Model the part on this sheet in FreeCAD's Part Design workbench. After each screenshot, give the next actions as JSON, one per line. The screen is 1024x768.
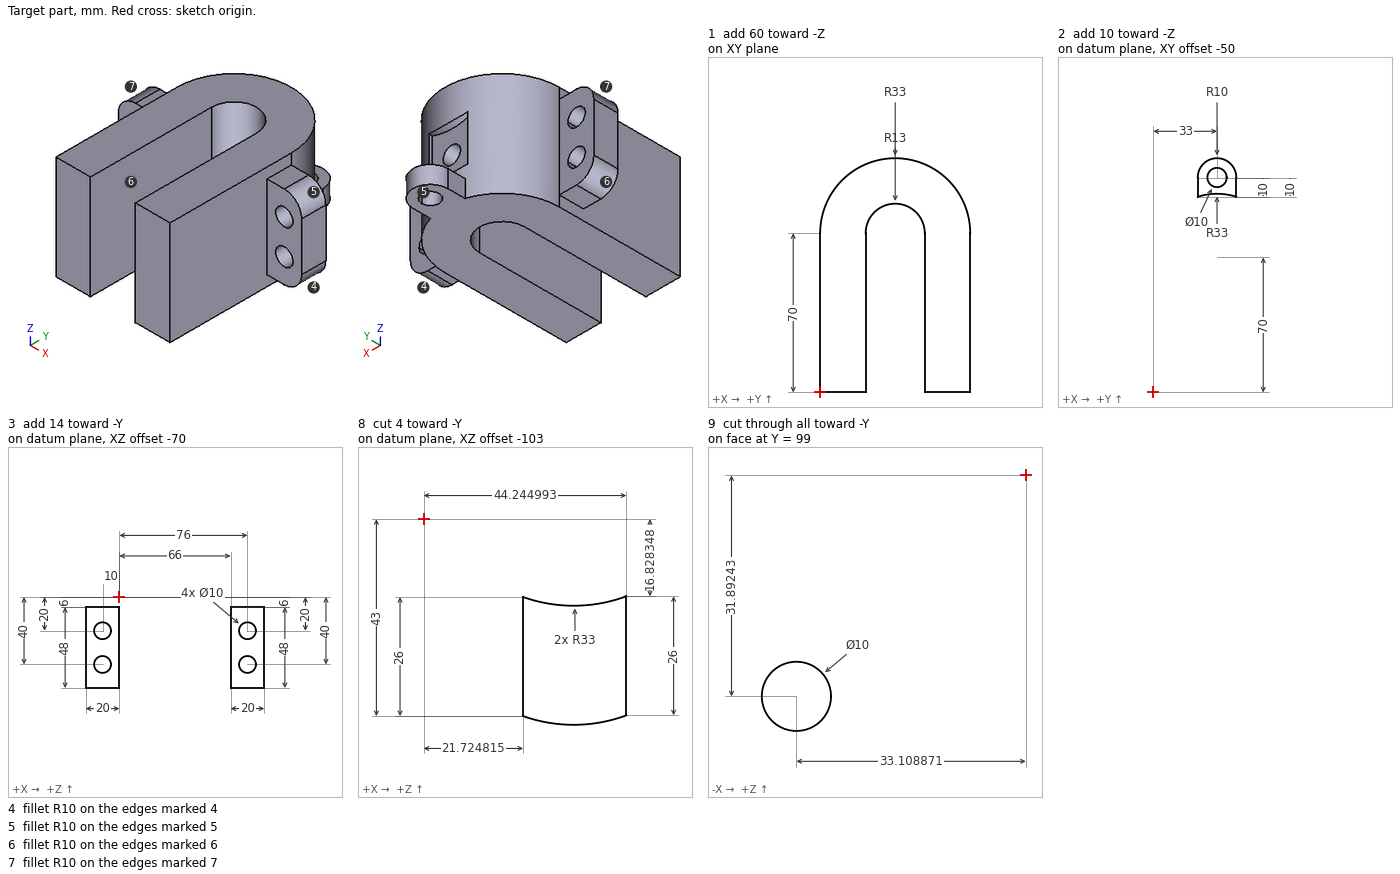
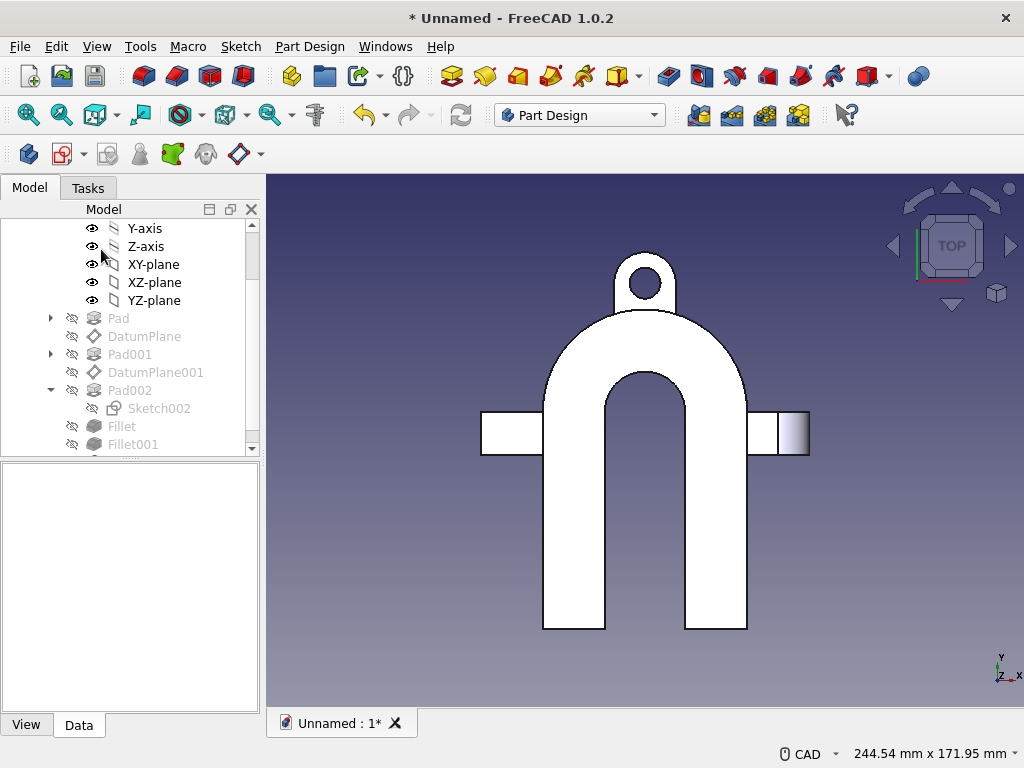
{"action": "left_click", "coordinate": [481, 432]}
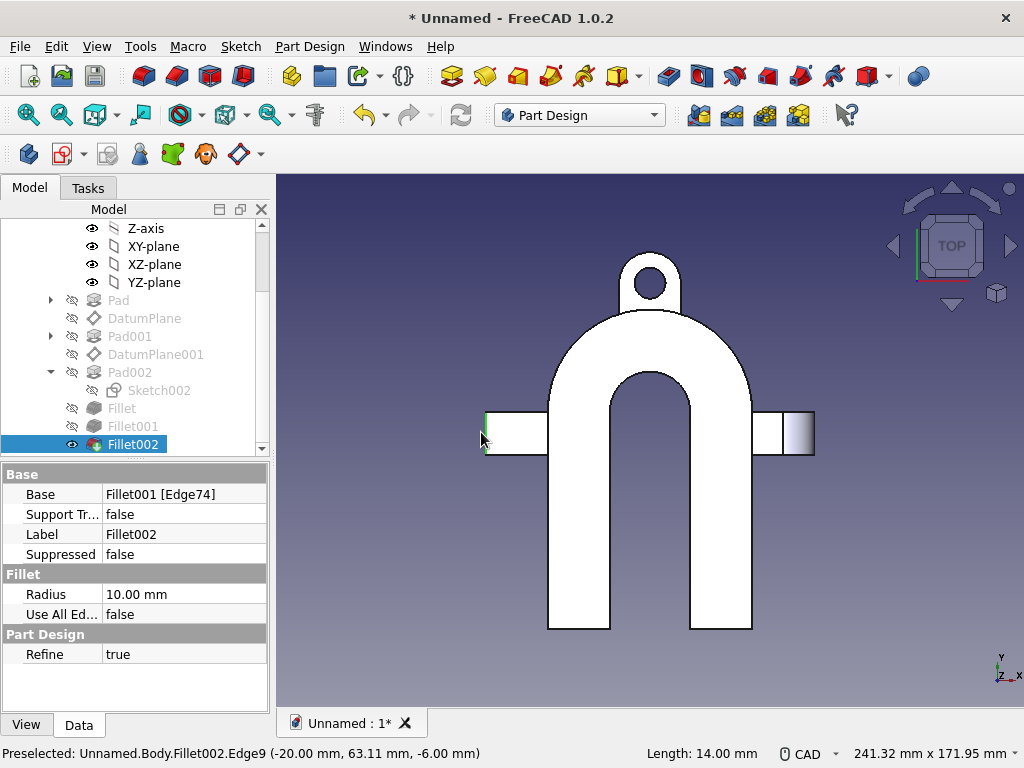
{"action": "left_click", "coordinate": [144, 76]}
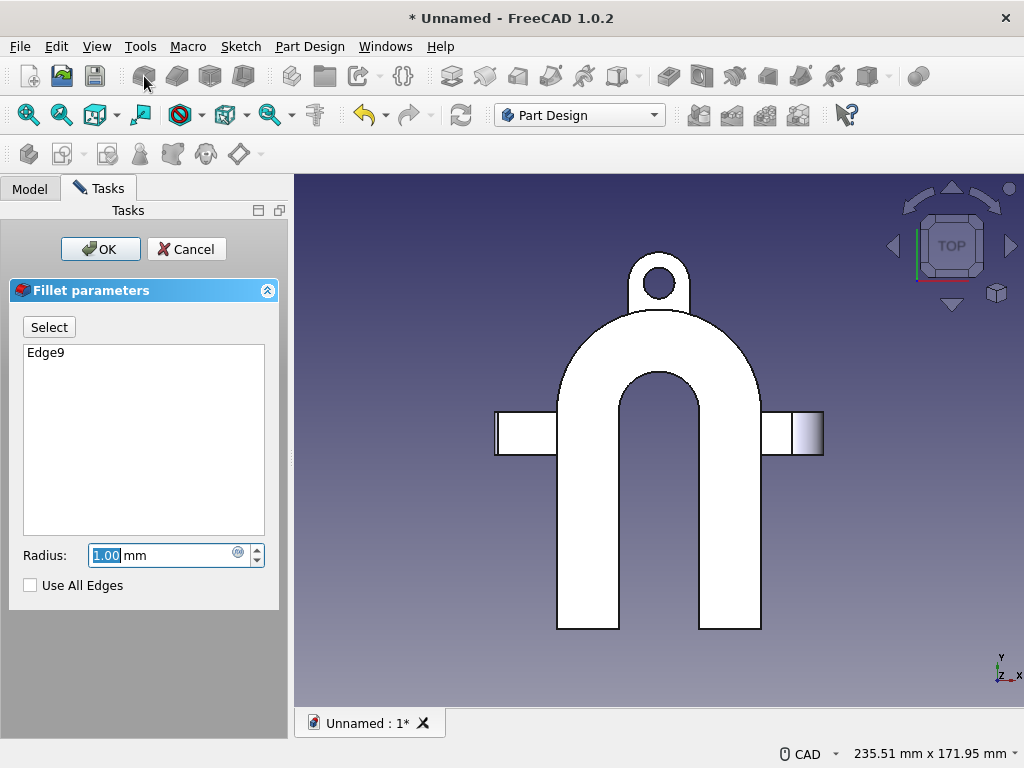
{"action": "type", "text": "10"}
{"action": "key", "text": "Tab"}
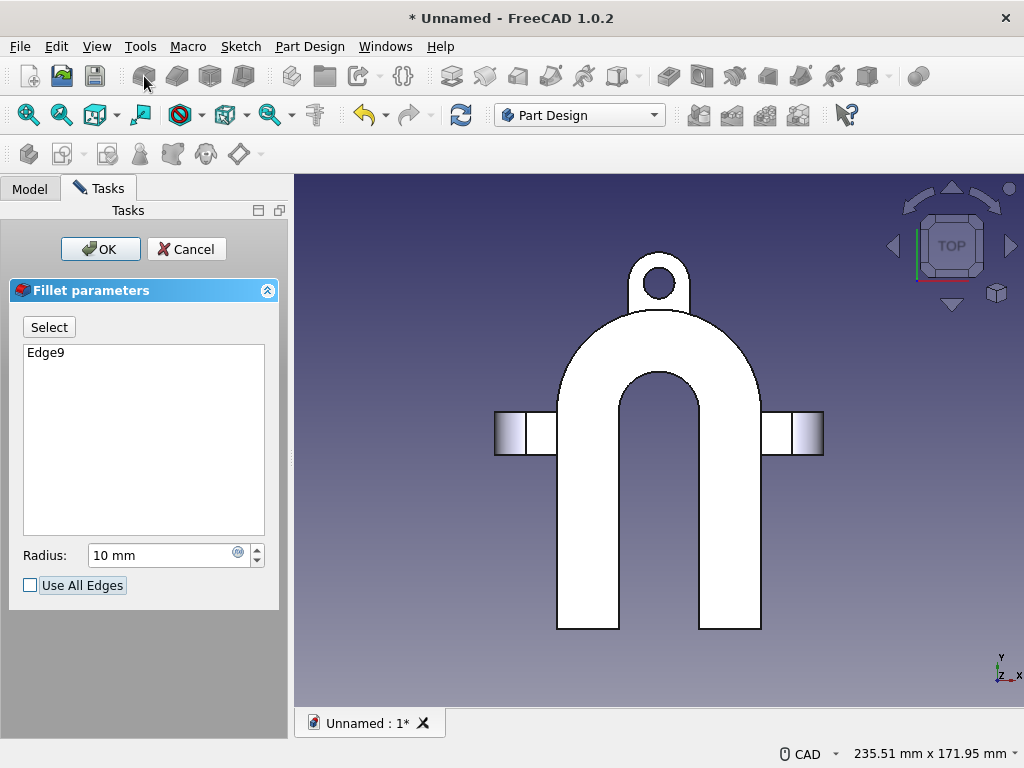
{"action": "left_click", "coordinate": [101, 249]}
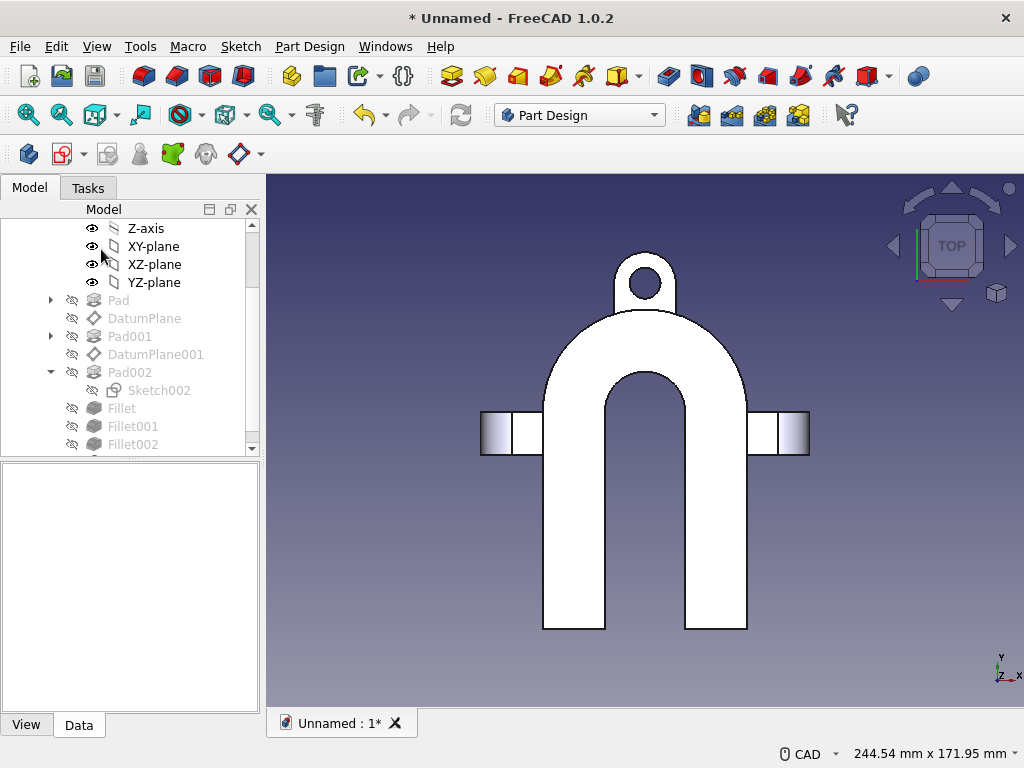
{"action": "scroll", "coordinate": [161, 332], "scroll_direction": "down", "scroll_amount": 3}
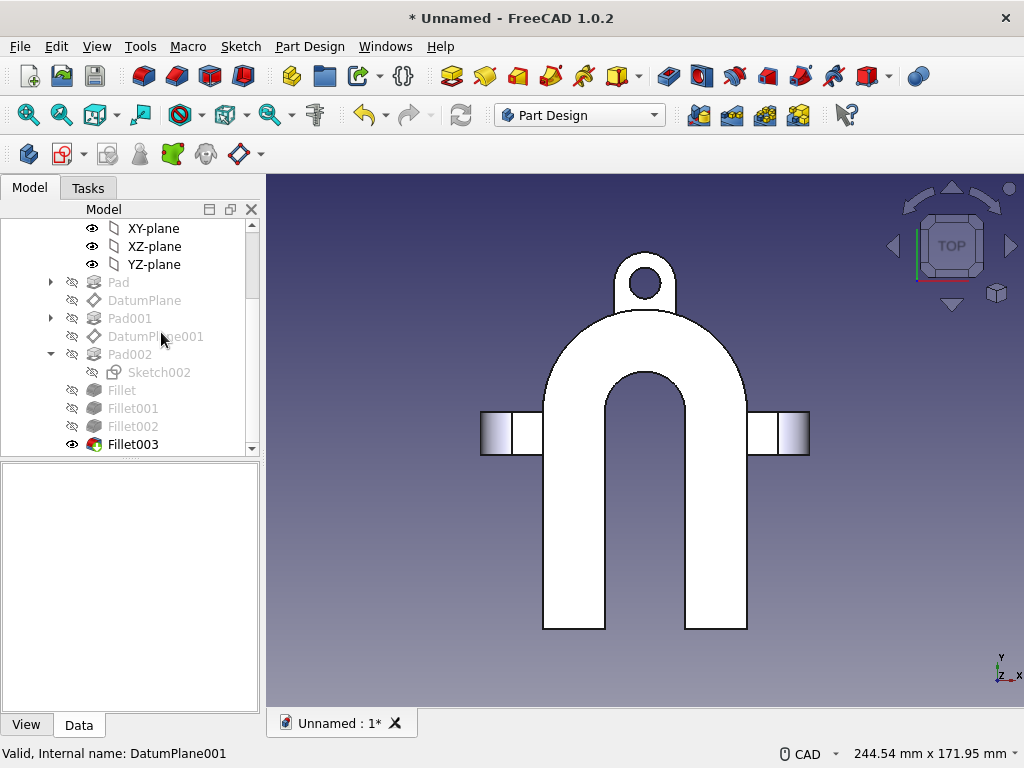
{"action": "scroll", "coordinate": [161, 332], "scroll_direction": "up", "scroll_amount": 15}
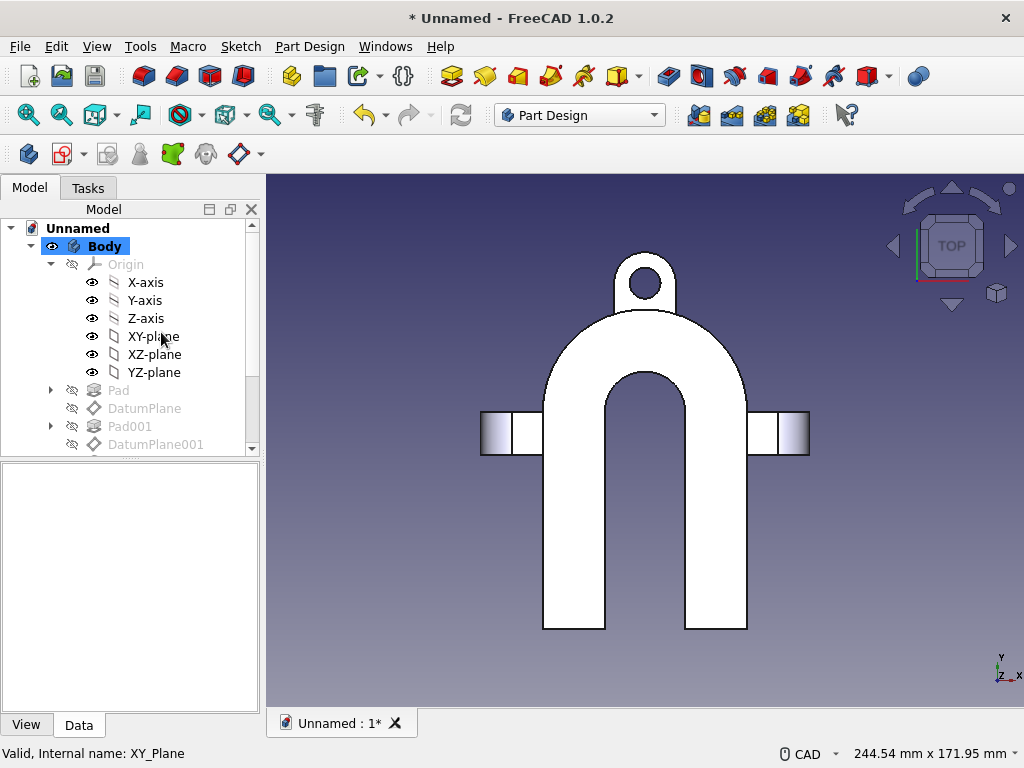
{"action": "left_click", "coordinate": [137, 354]}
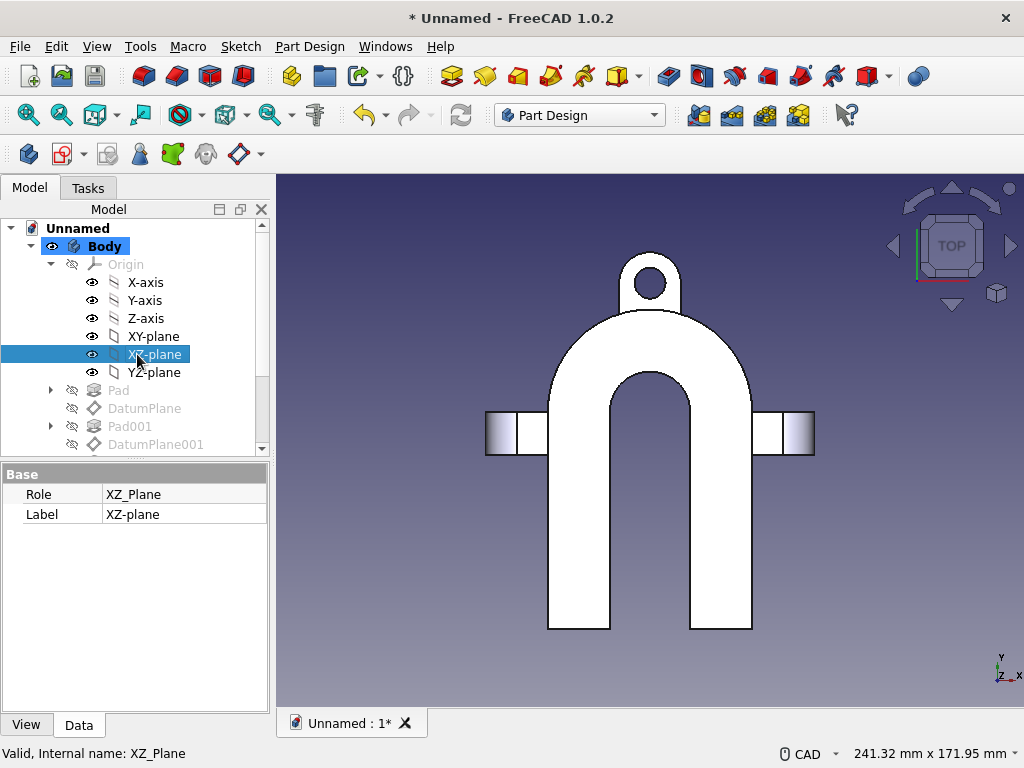
{"action": "left_click", "coordinate": [238, 154]}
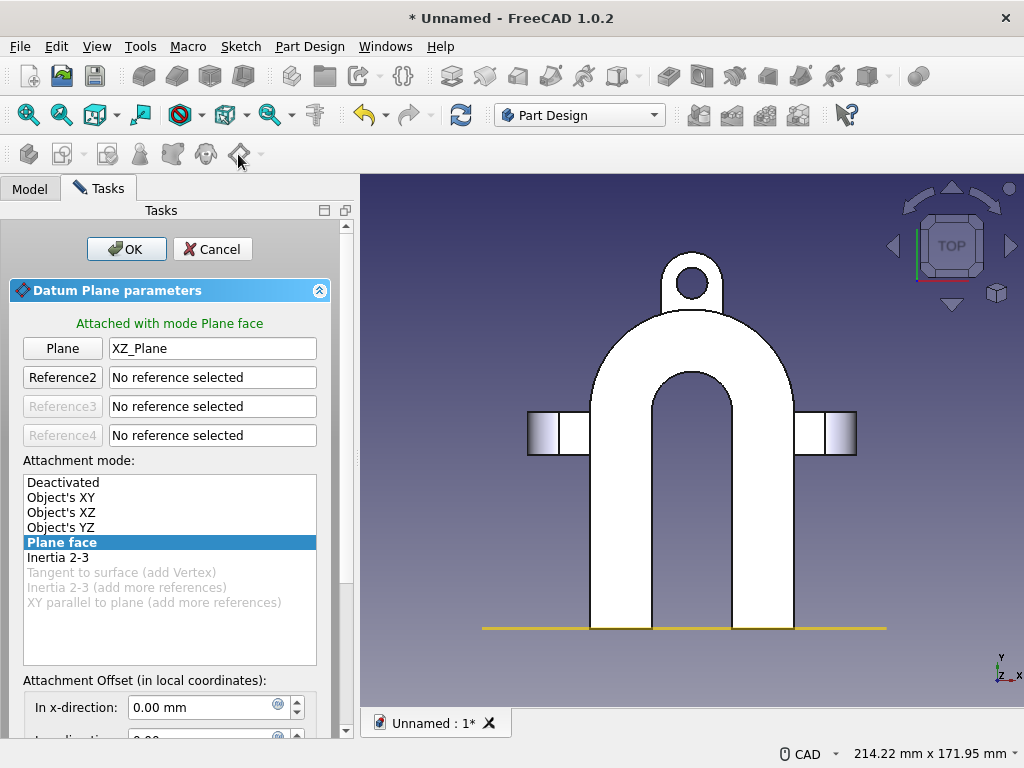
{"action": "scroll", "coordinate": [346, 479], "scroll_direction": "down", "scroll_amount": 2}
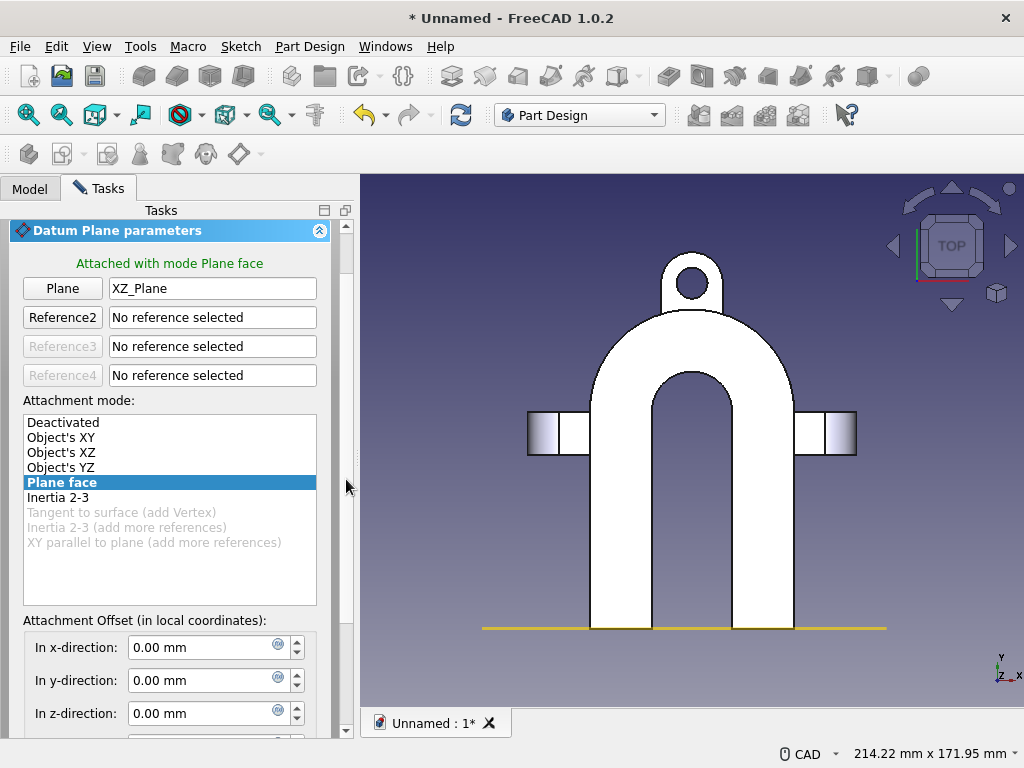
{"action": "triple_click", "coordinate": [210, 654]}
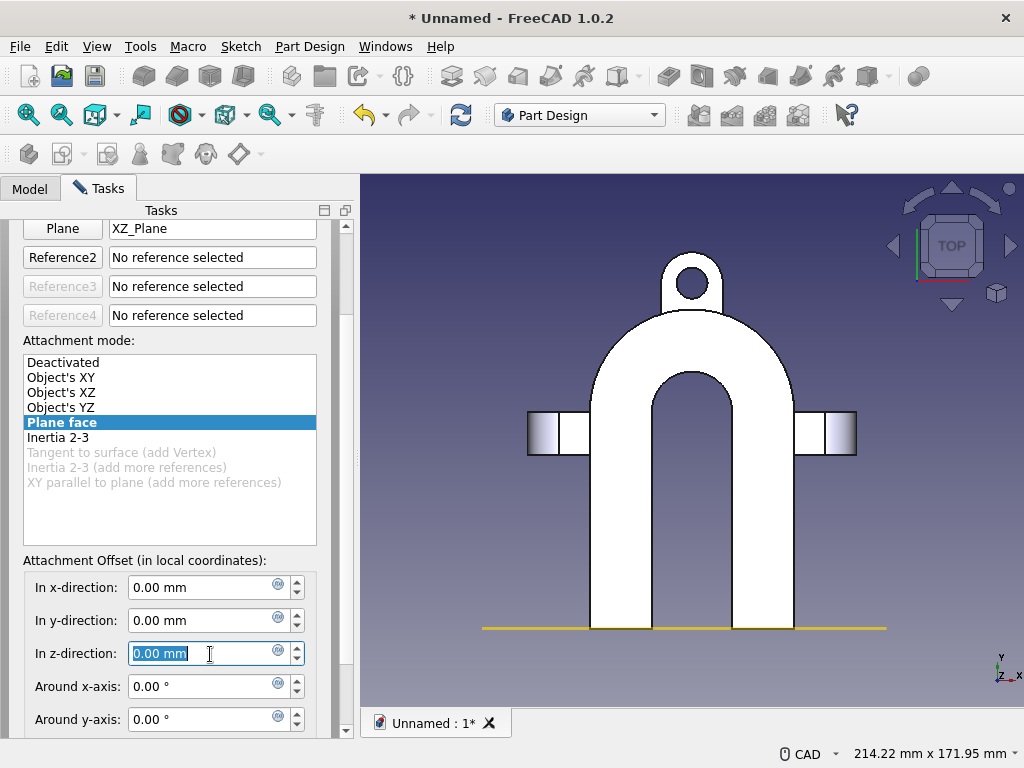
{"action": "type", "text": "-103"}
{"action": "key", "text": "Tab"}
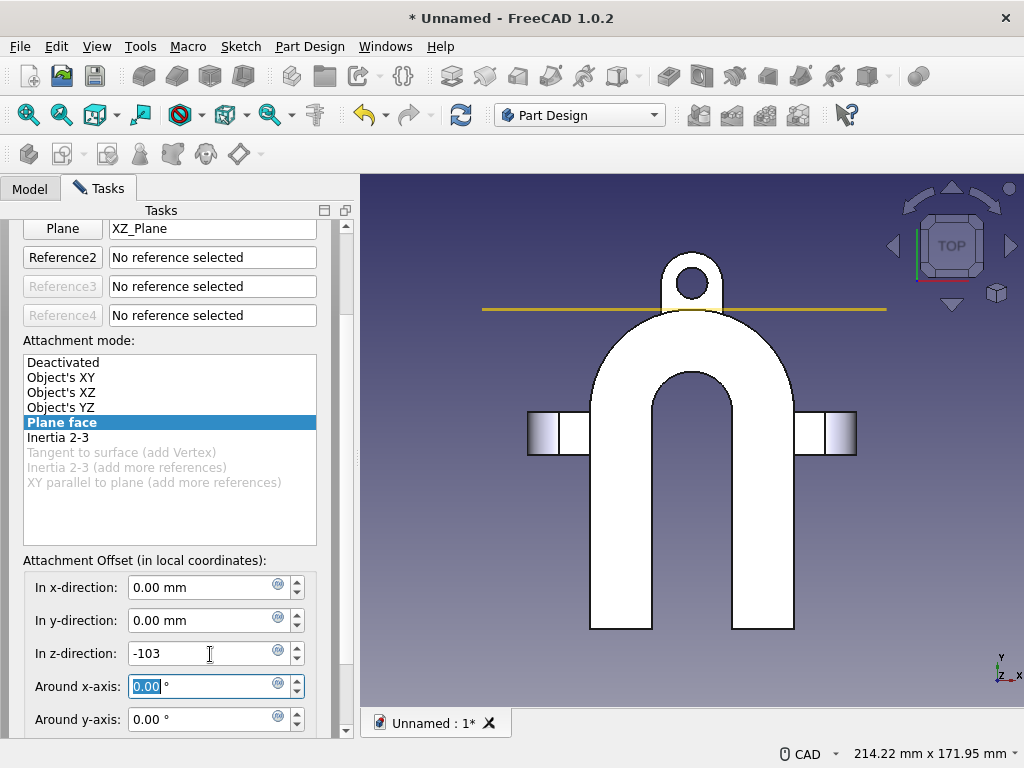
{"action": "scroll", "coordinate": [346, 479], "scroll_direction": "up", "scroll_amount": 3}